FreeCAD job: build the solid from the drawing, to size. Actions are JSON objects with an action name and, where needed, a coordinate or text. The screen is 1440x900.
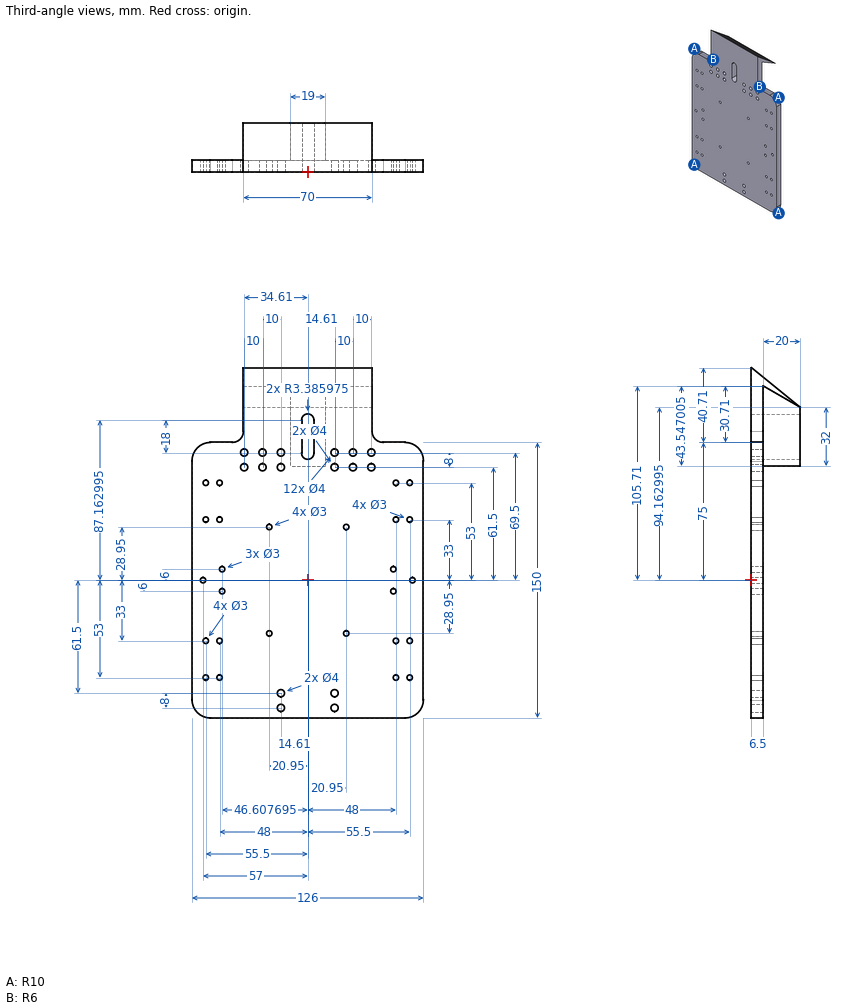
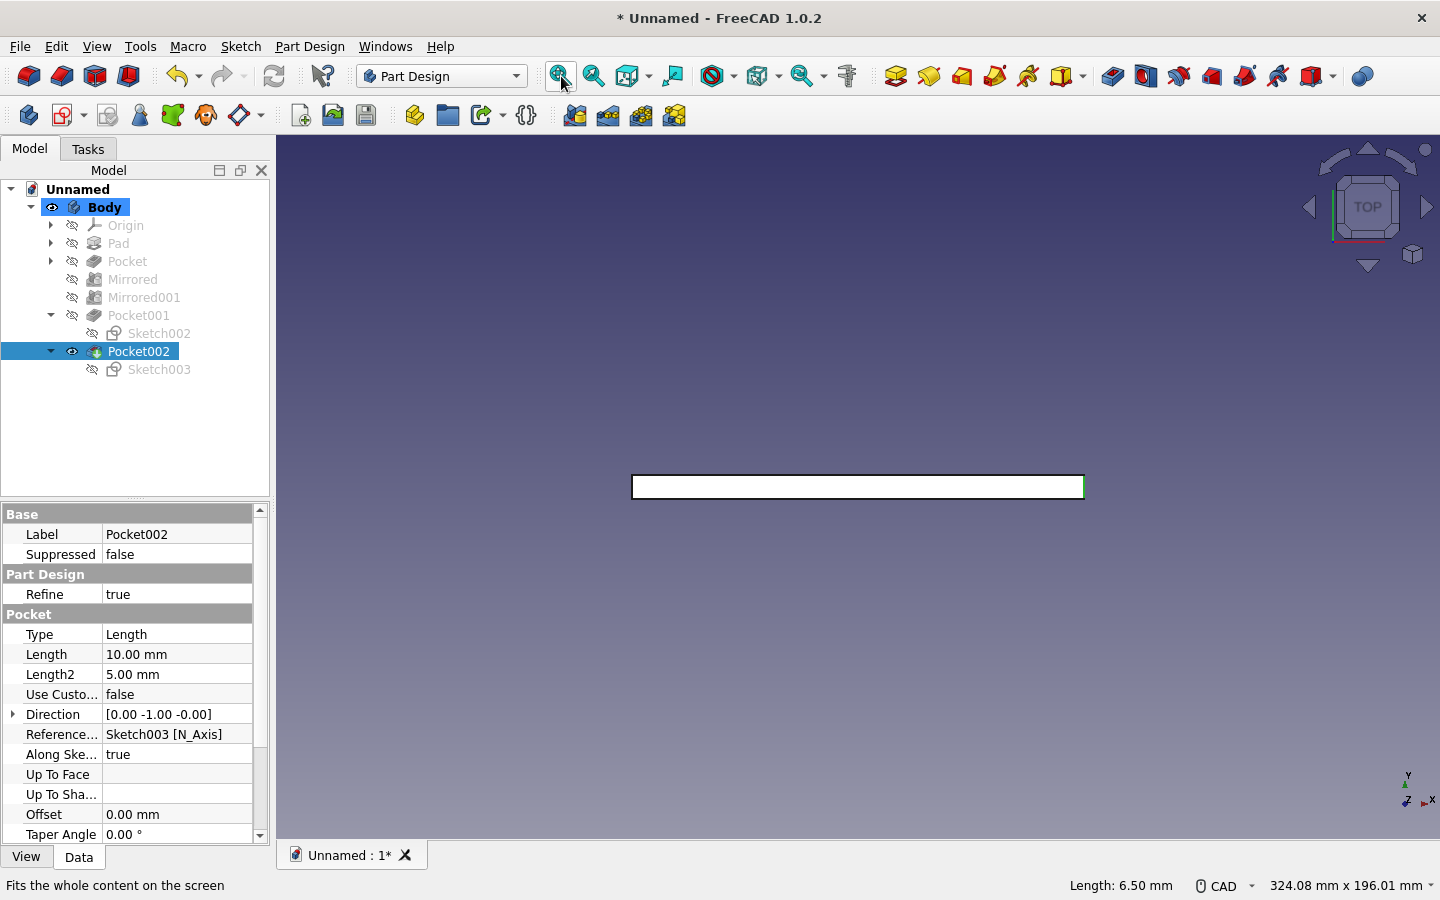
{"action": "left_click", "coordinate": [632, 486], "text": "ctrl"}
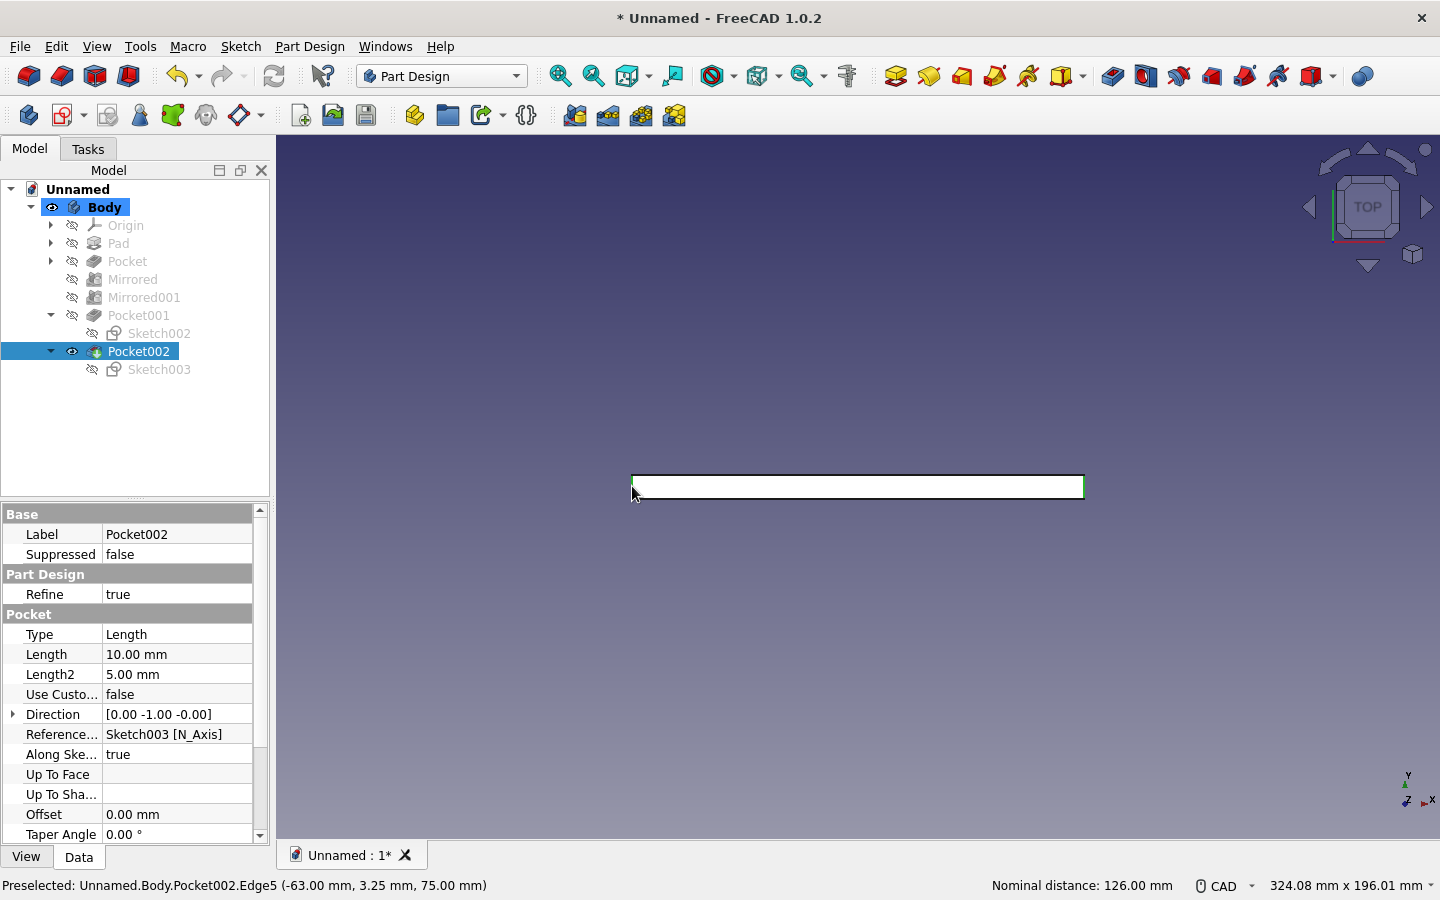
{"action": "key", "text": "1"}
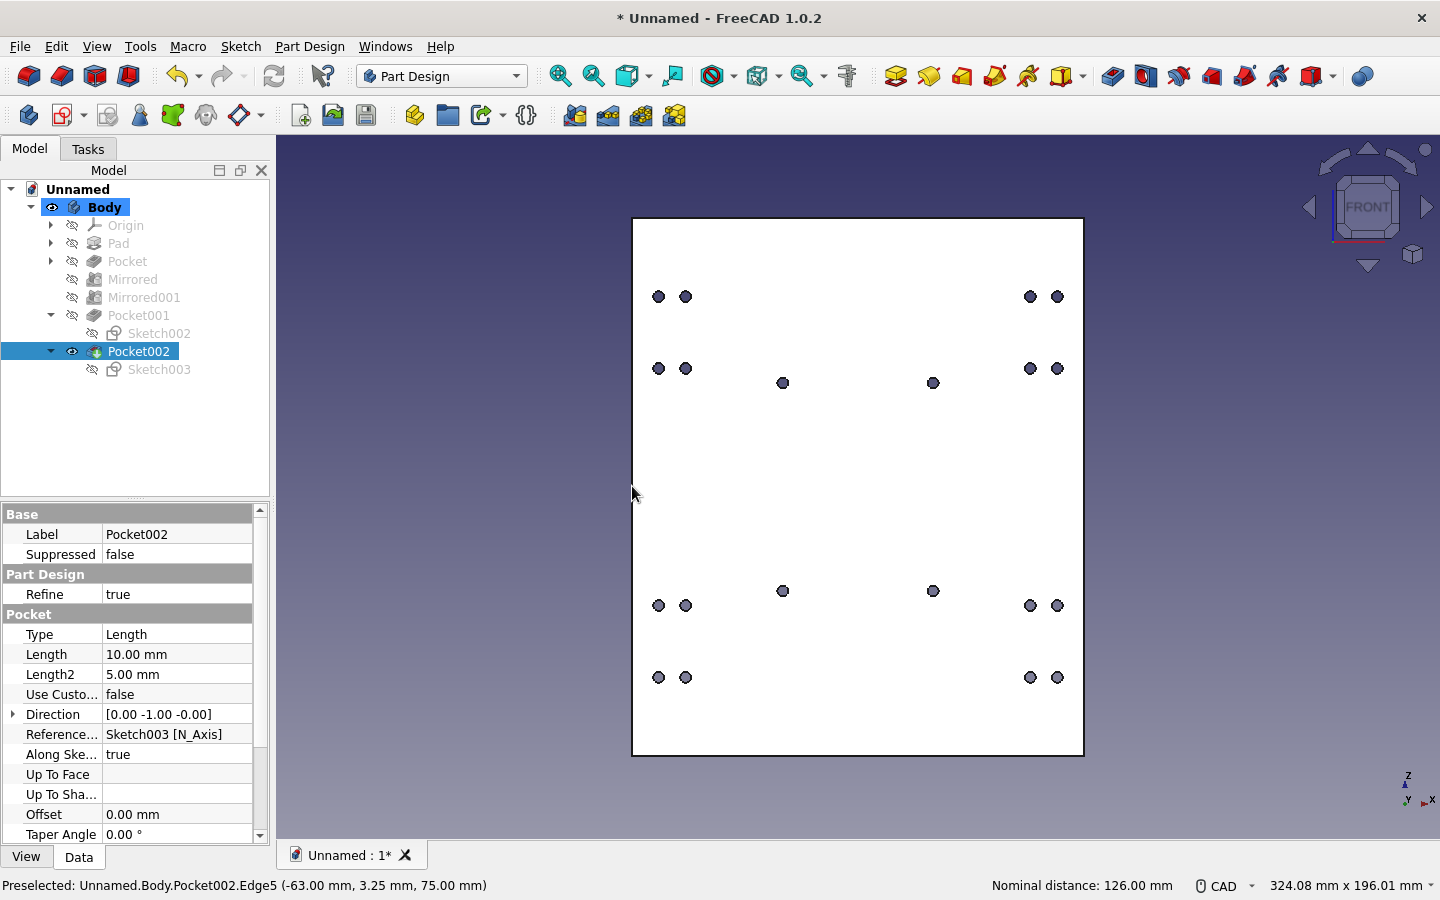
{"action": "key", "text": "3"}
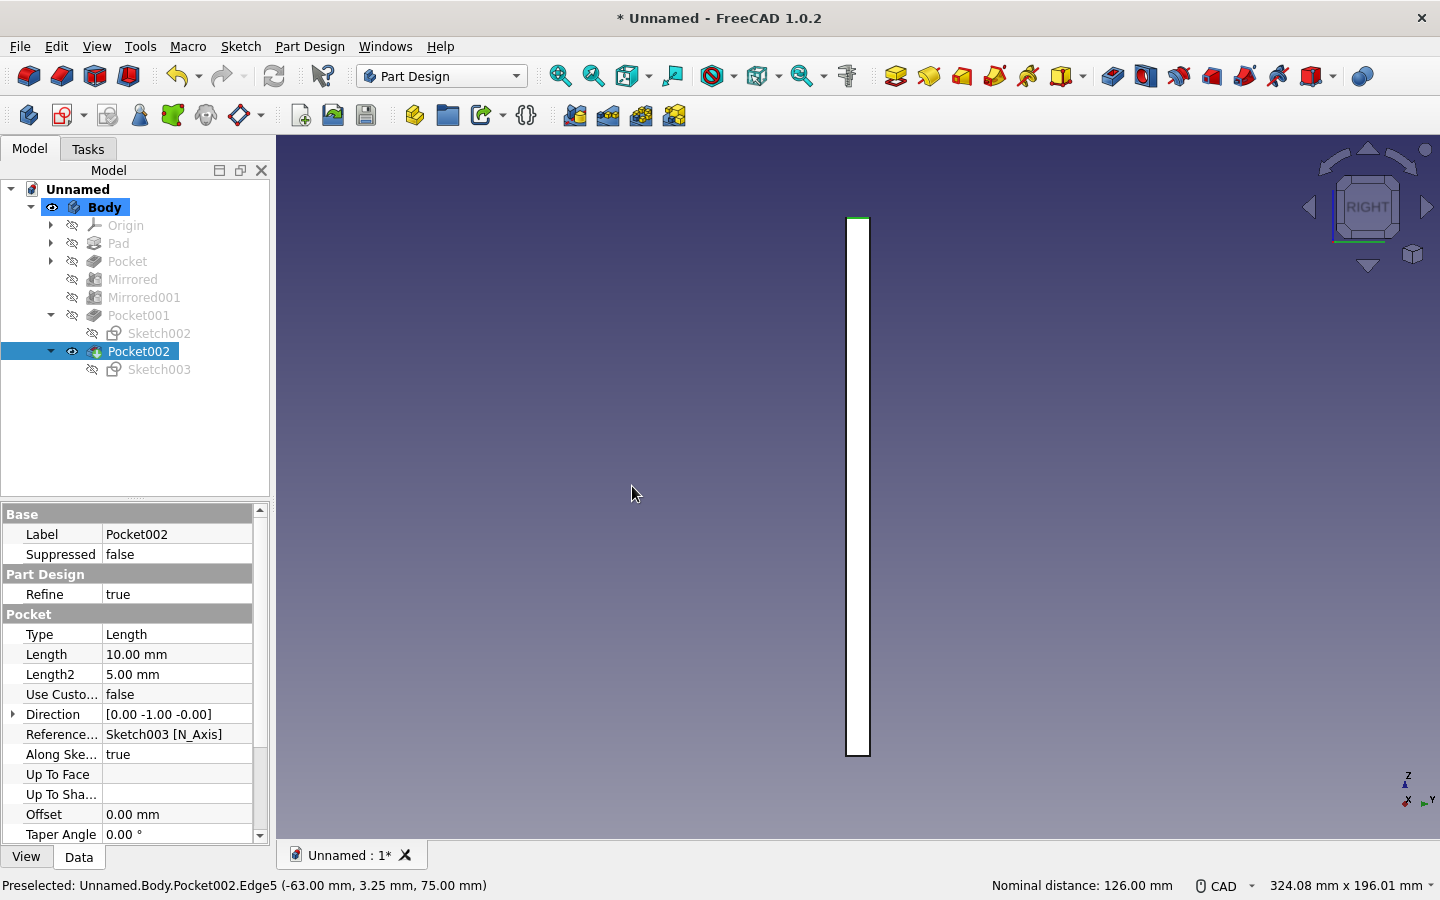
{"action": "left_click", "coordinate": [858, 755], "text": "ctrl"}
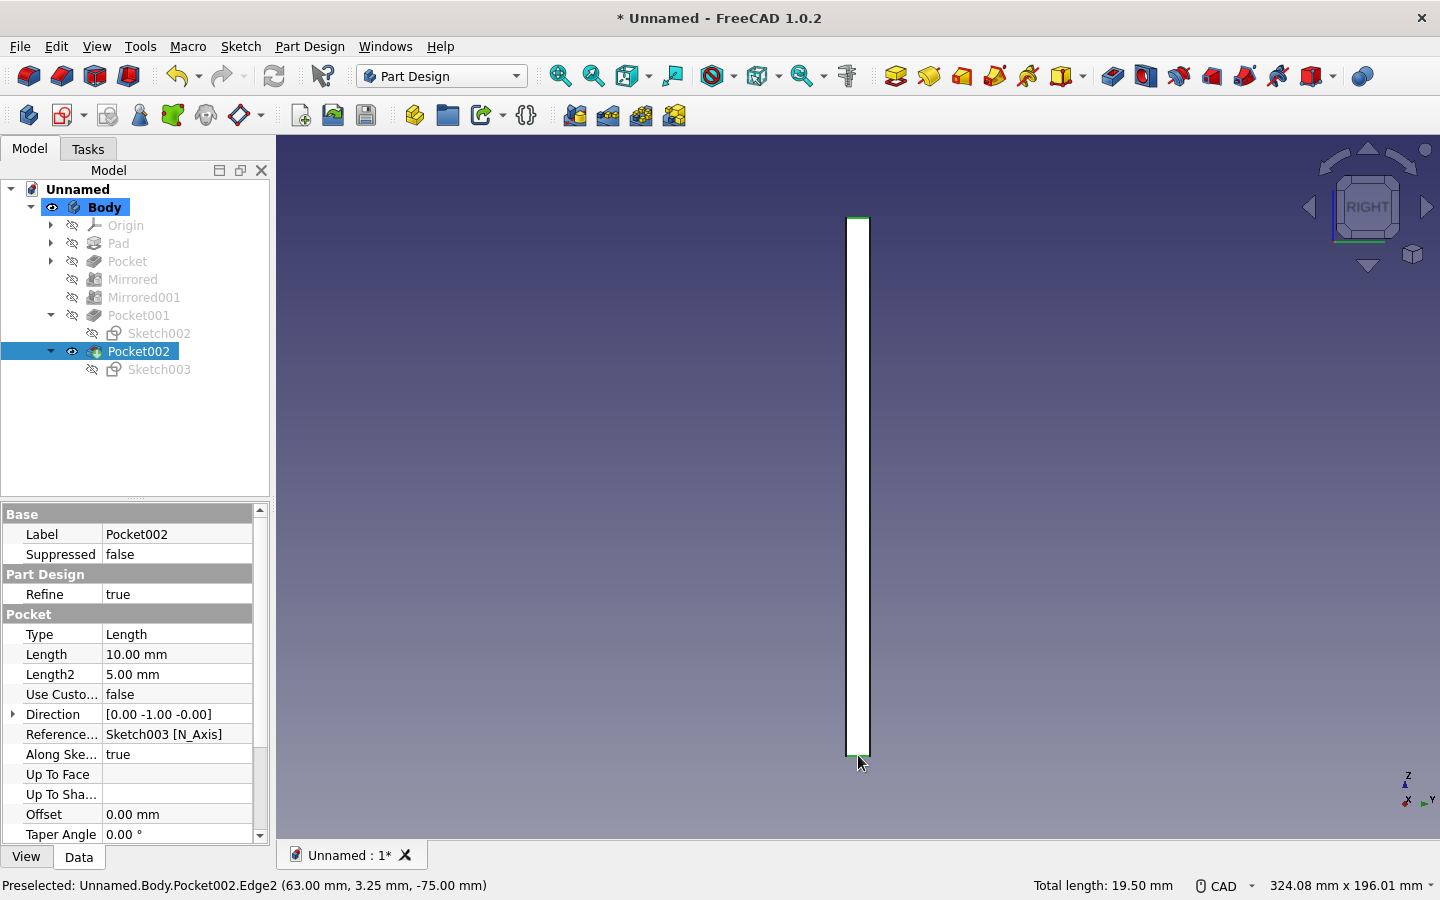
{"action": "key", "text": "5"}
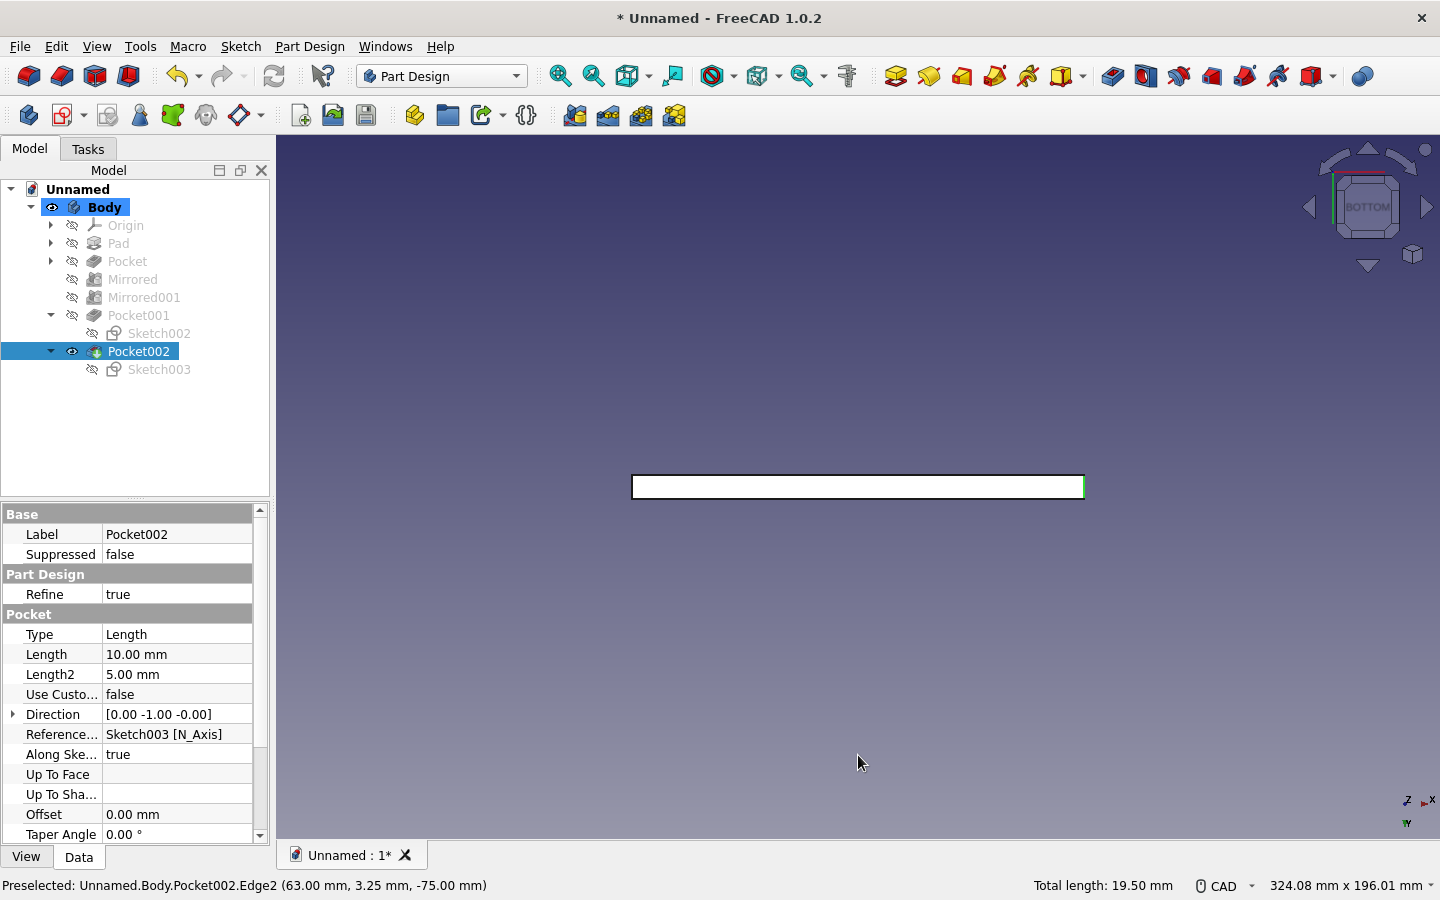
{"action": "left_click", "coordinate": [561, 76]}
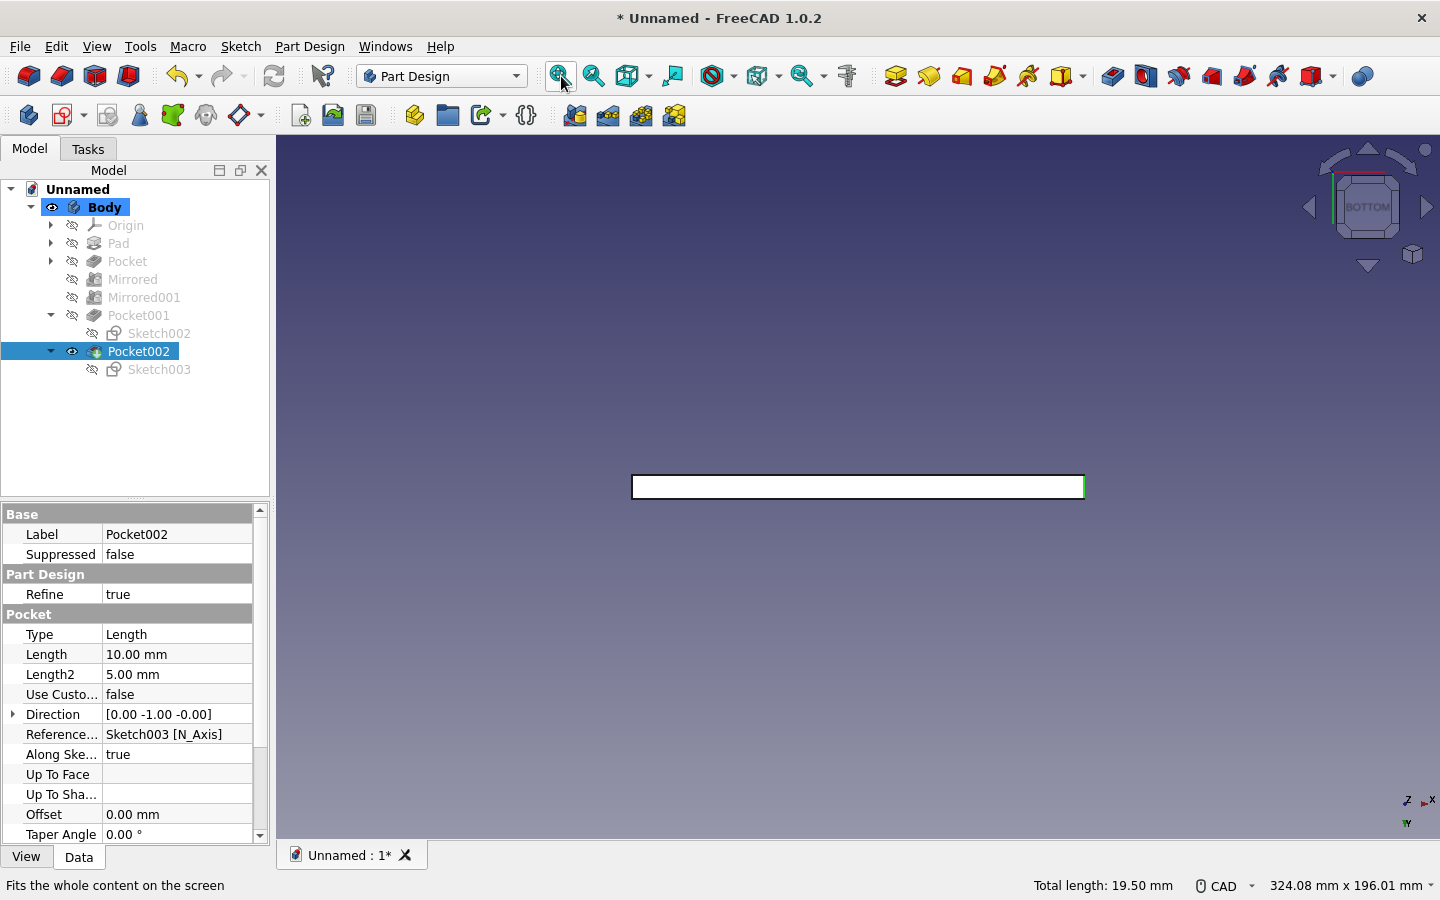
{"action": "left_click", "coordinate": [632, 486], "text": "ctrl"}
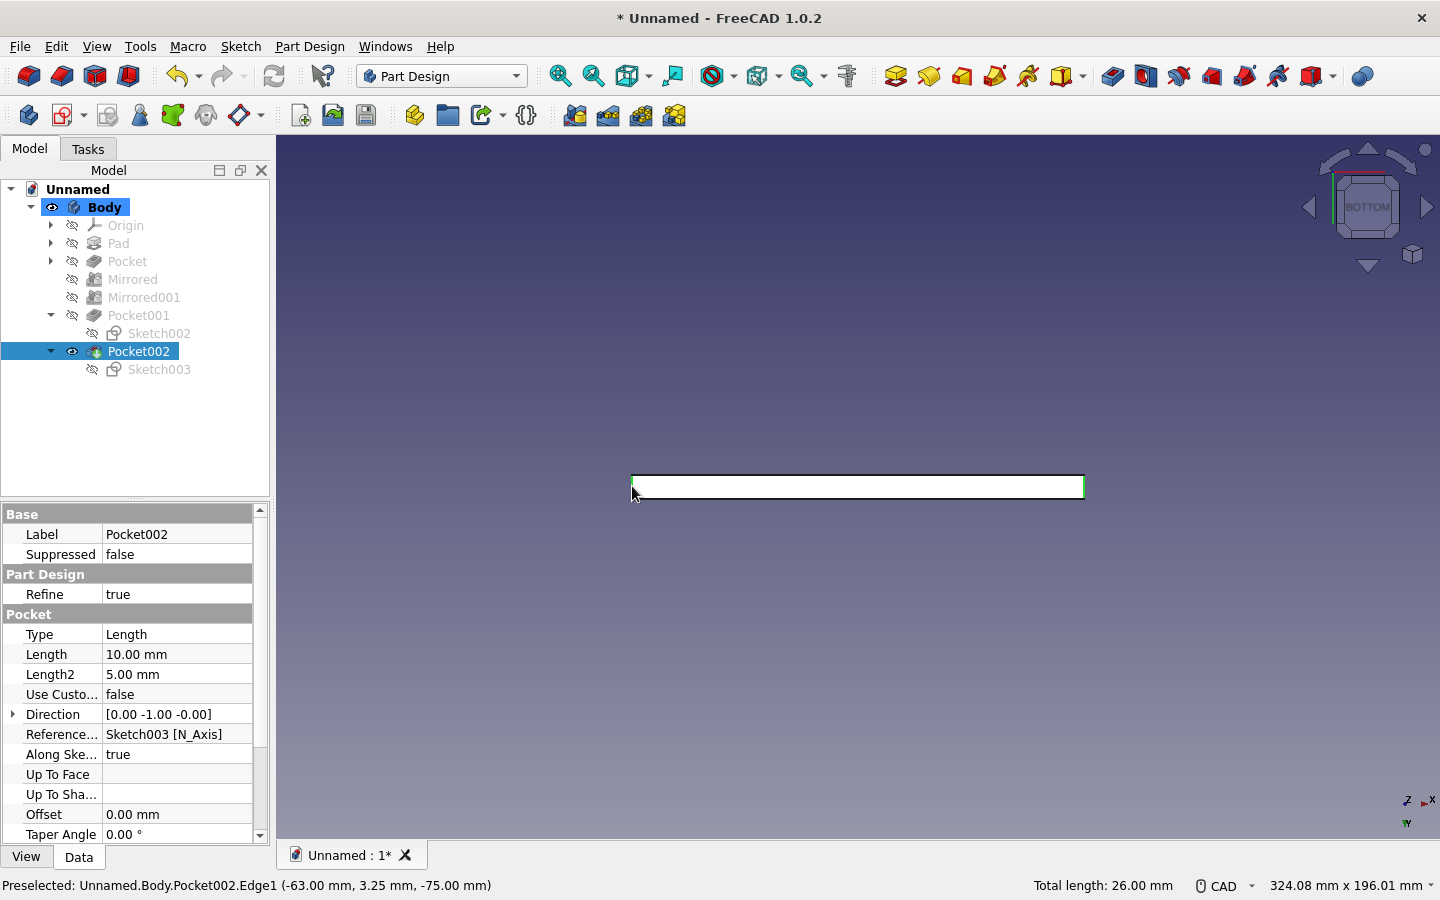
{"action": "left_click", "coordinate": [29, 76]}